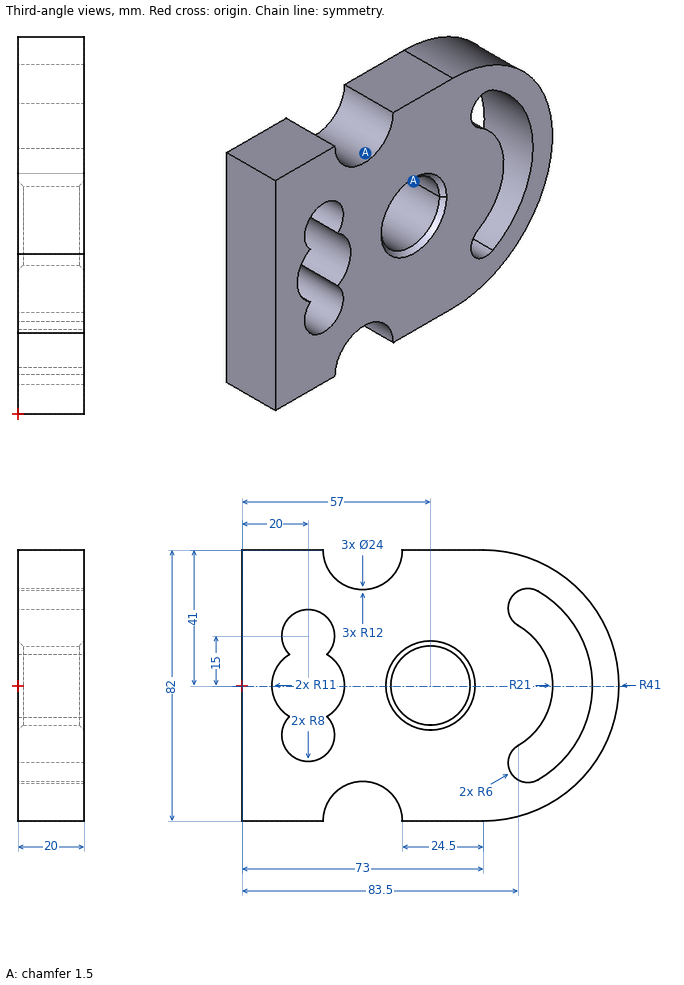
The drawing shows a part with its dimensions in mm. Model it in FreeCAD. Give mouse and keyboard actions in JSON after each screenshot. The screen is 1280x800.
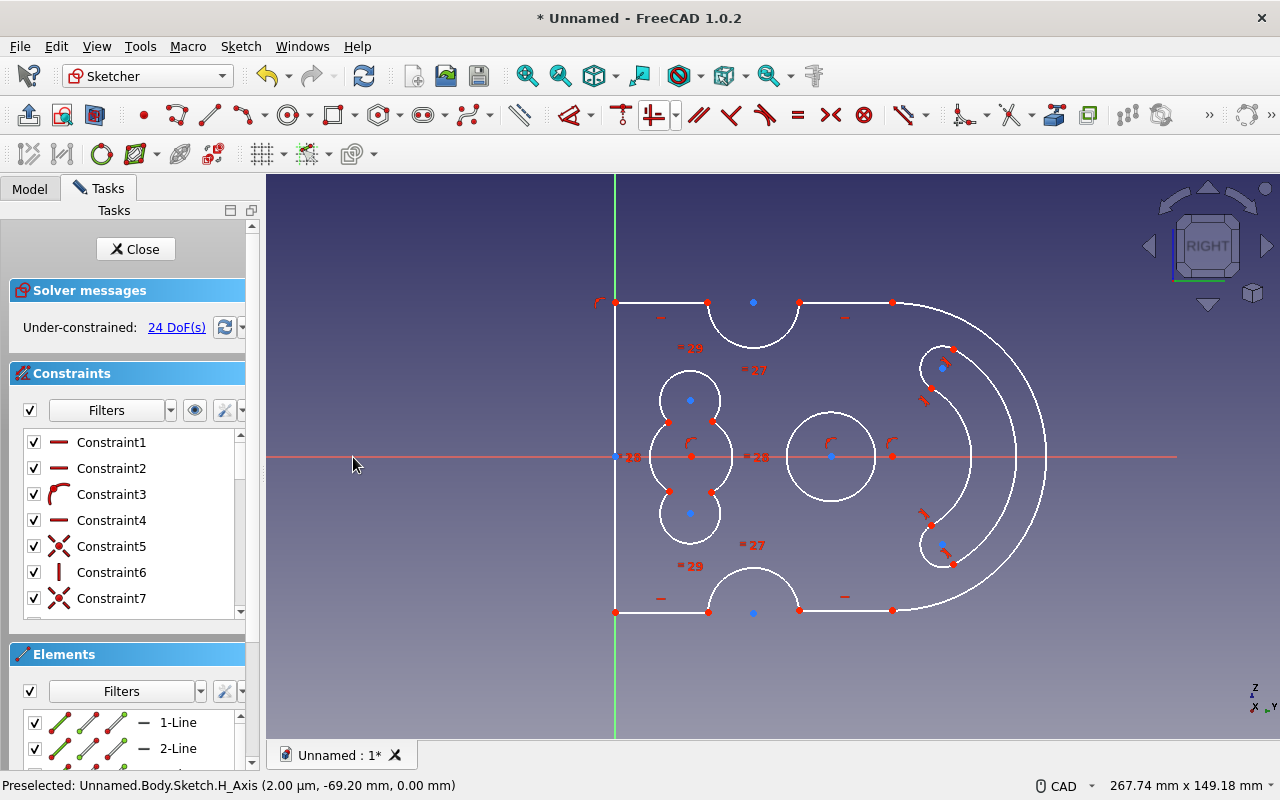
{"action": "left_click", "coordinate": [754, 303]}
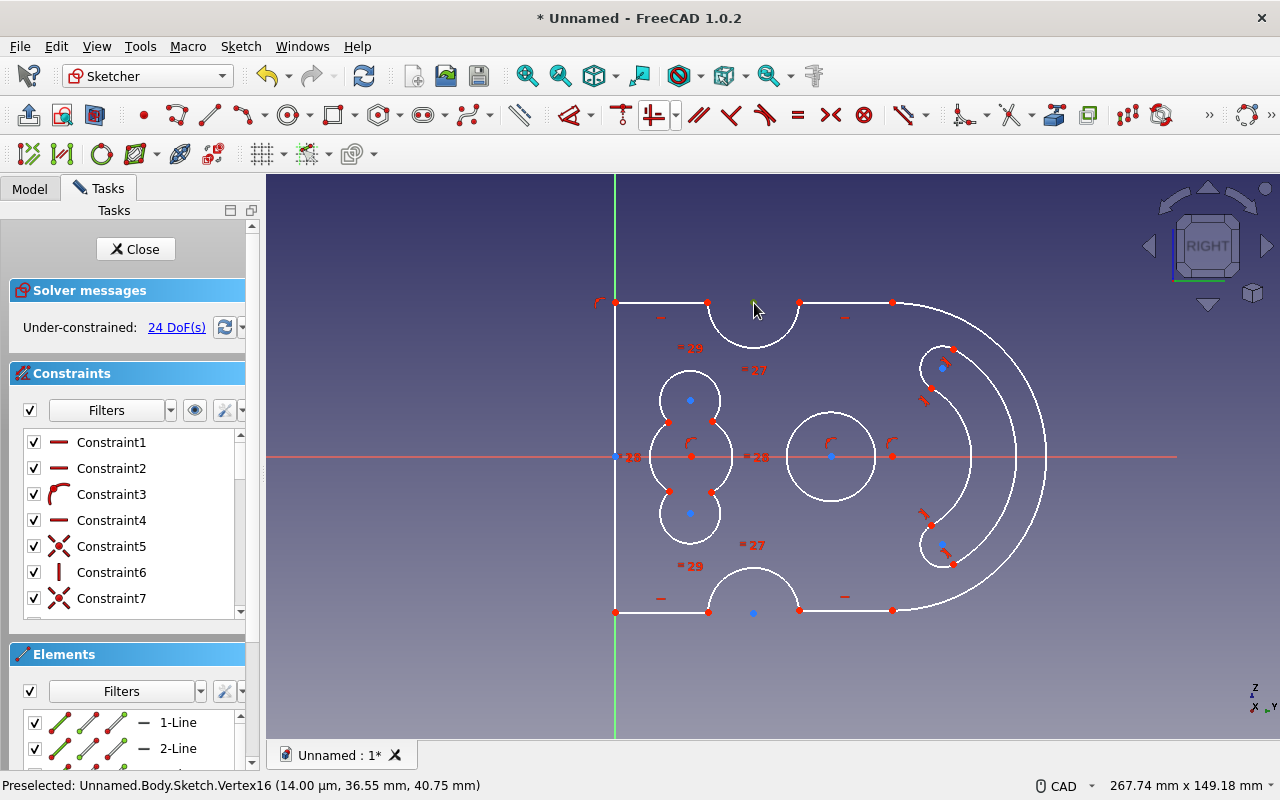
{"action": "left_click", "coordinate": [754, 614]}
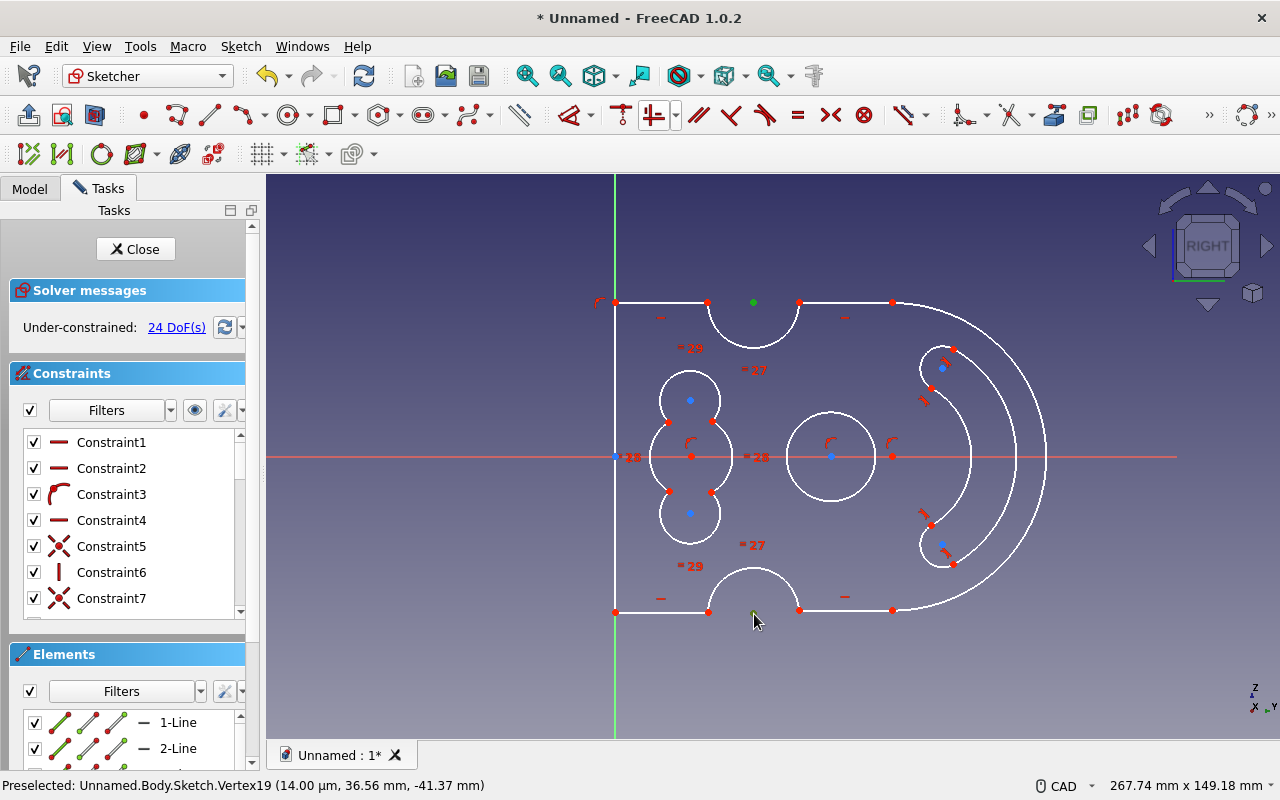
{"action": "left_click", "coordinate": [353, 457]}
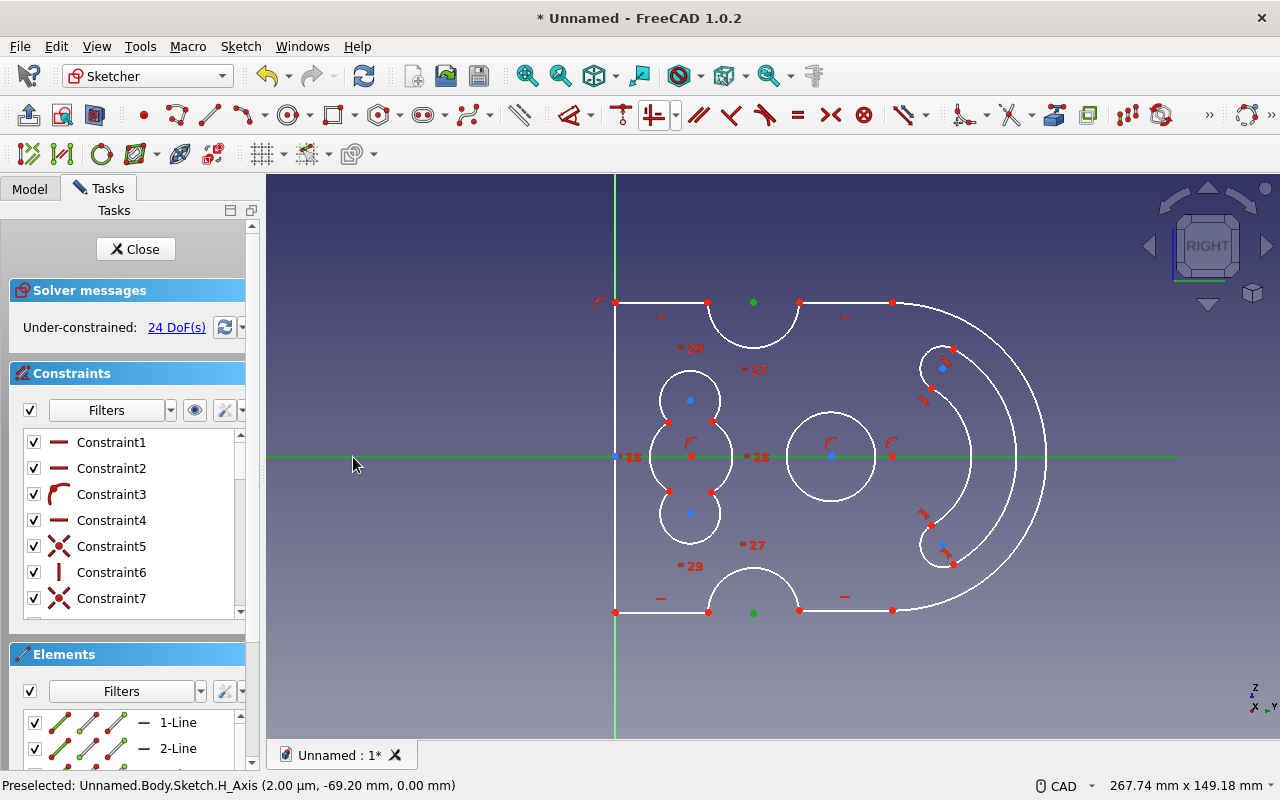
{"action": "left_click", "coordinate": [831, 116]}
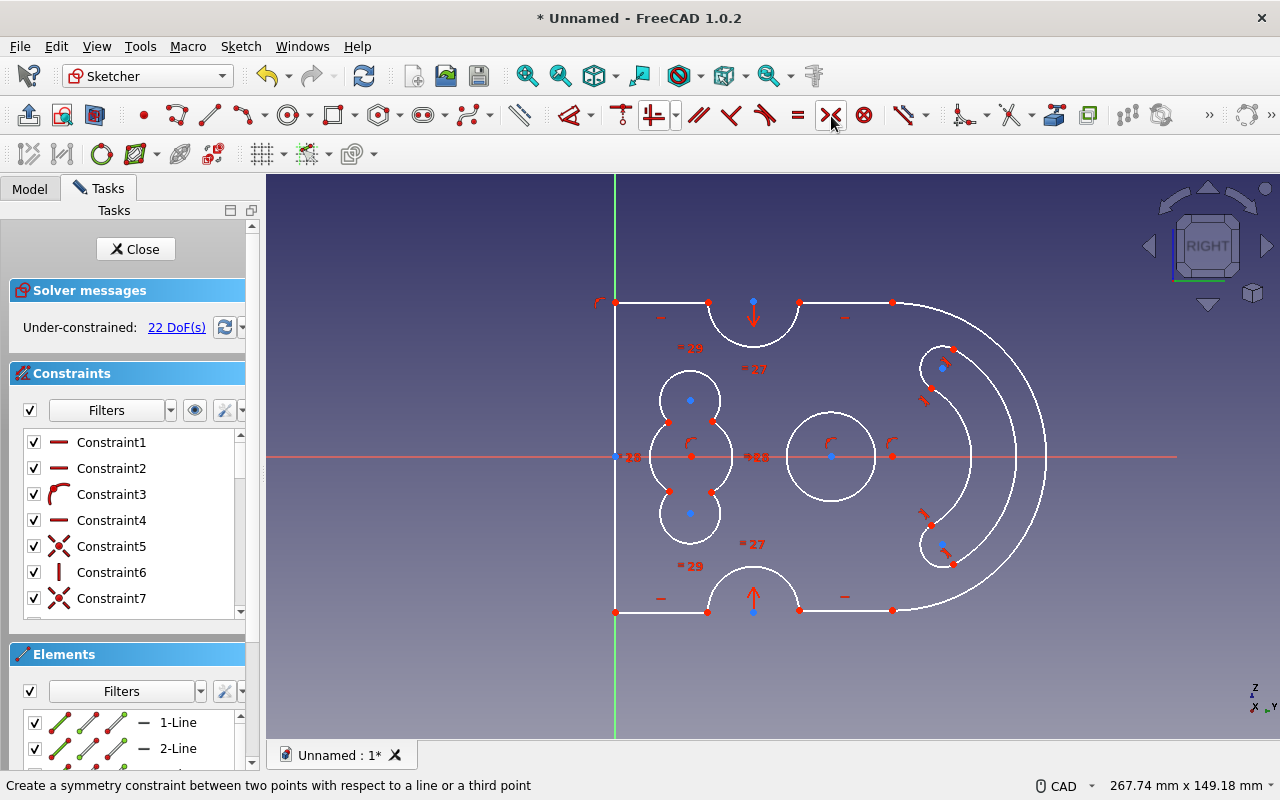
{"action": "left_click", "coordinate": [690, 401]}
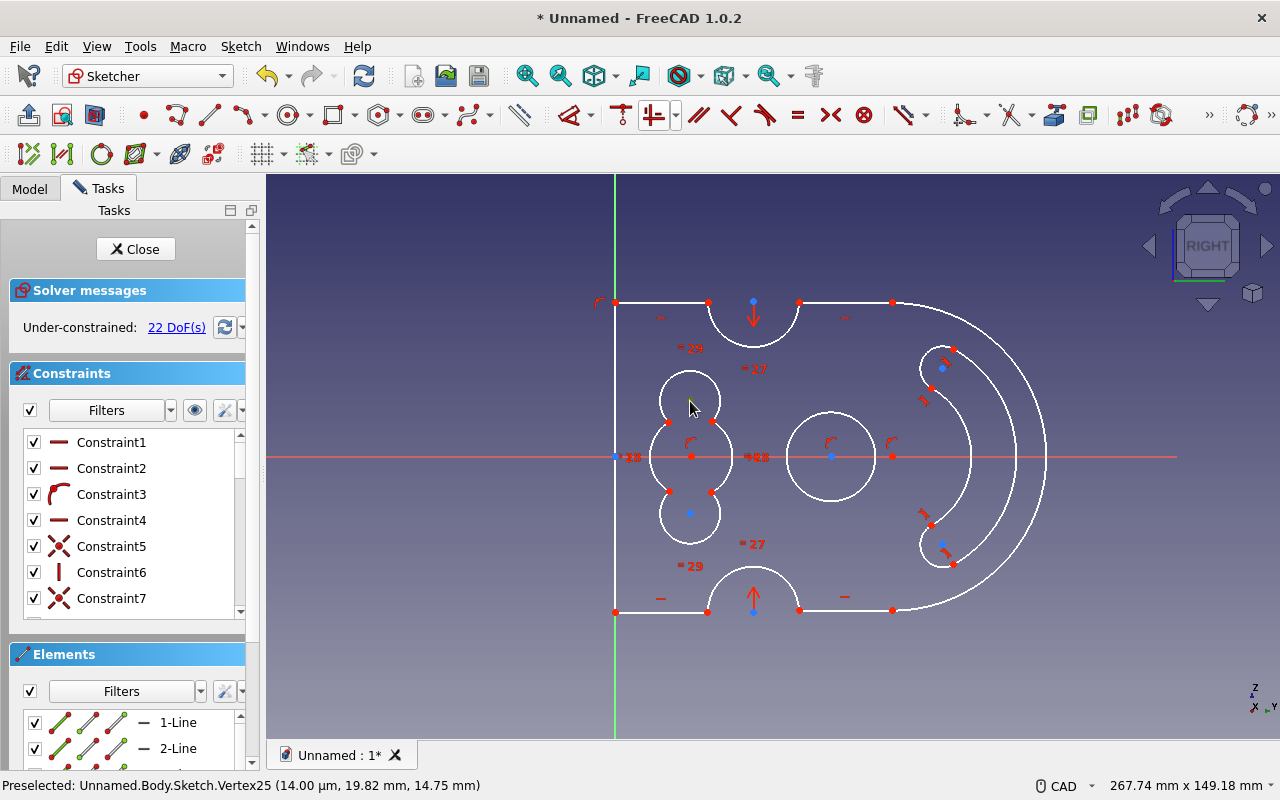
{"action": "left_click", "coordinate": [690, 514]}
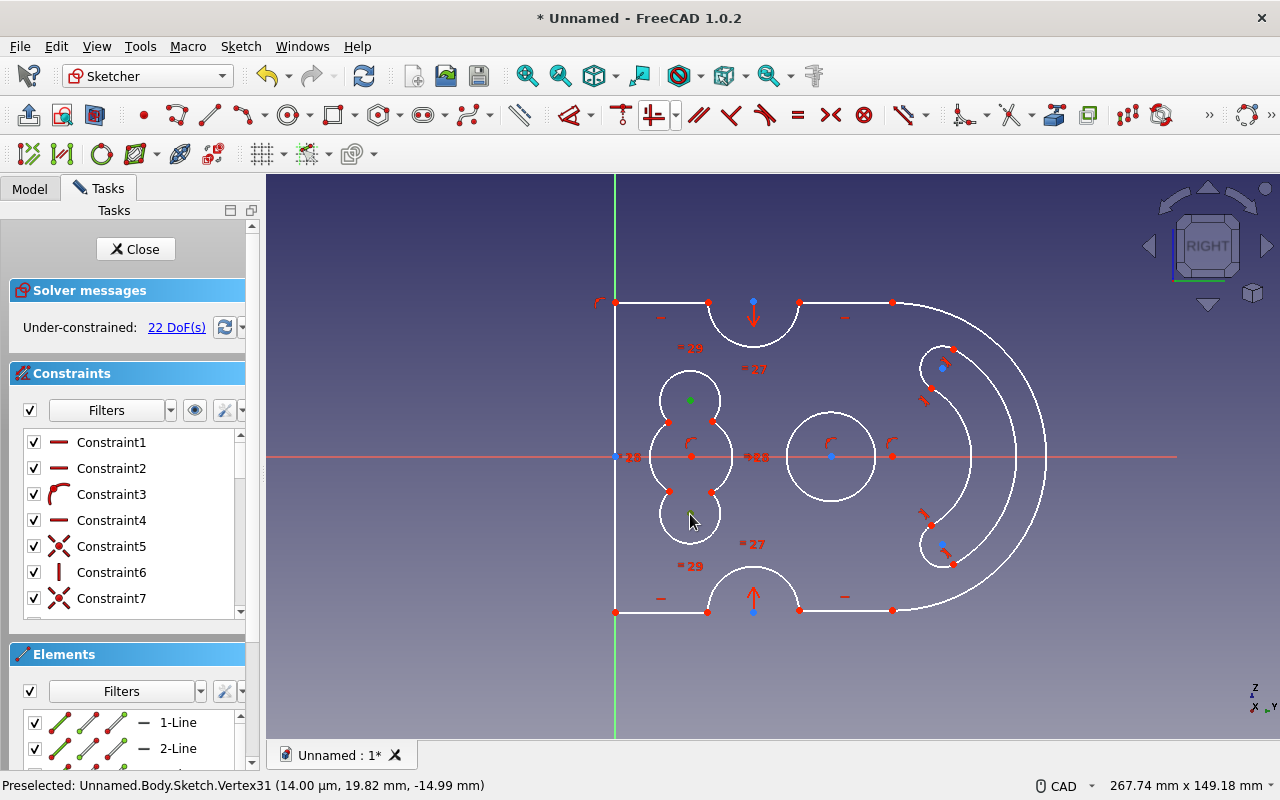
{"action": "left_click", "coordinate": [353, 457]}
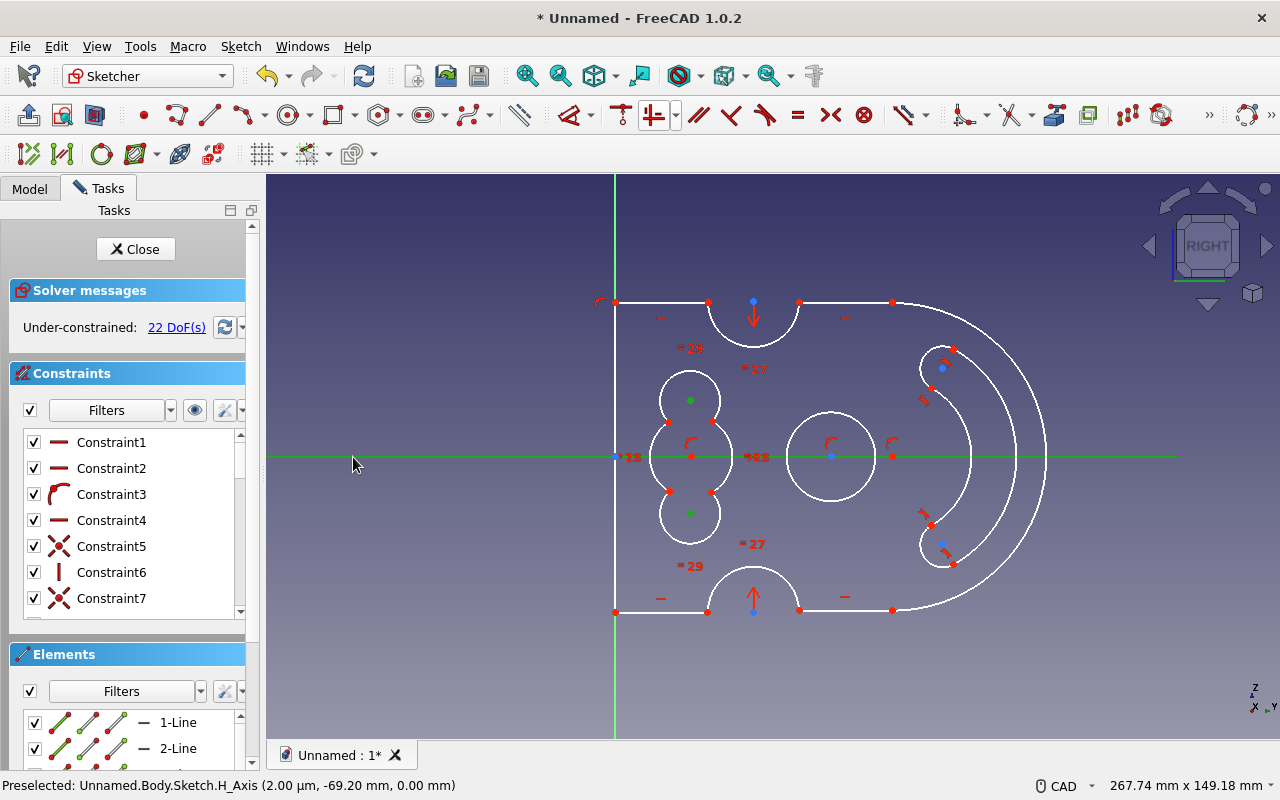
{"action": "key", "text": "s"}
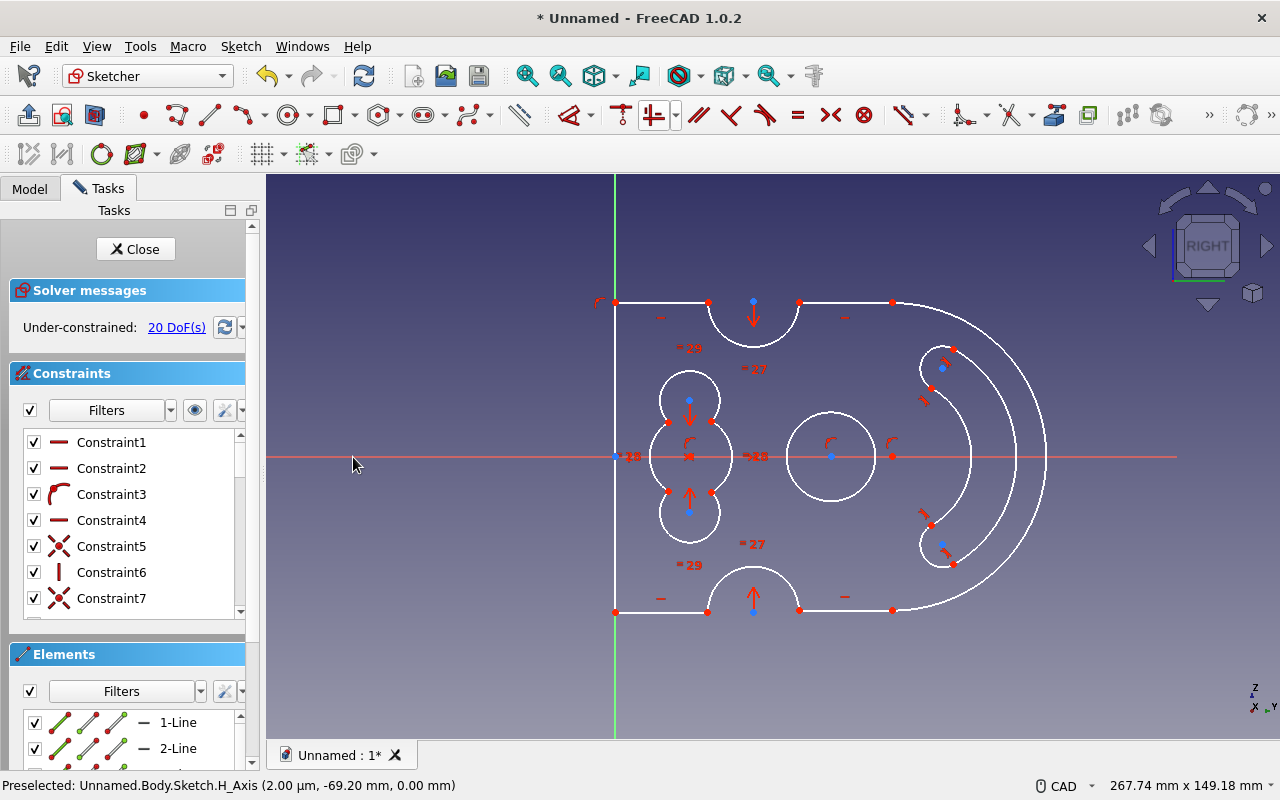
{"action": "left_click", "coordinate": [1017, 547]}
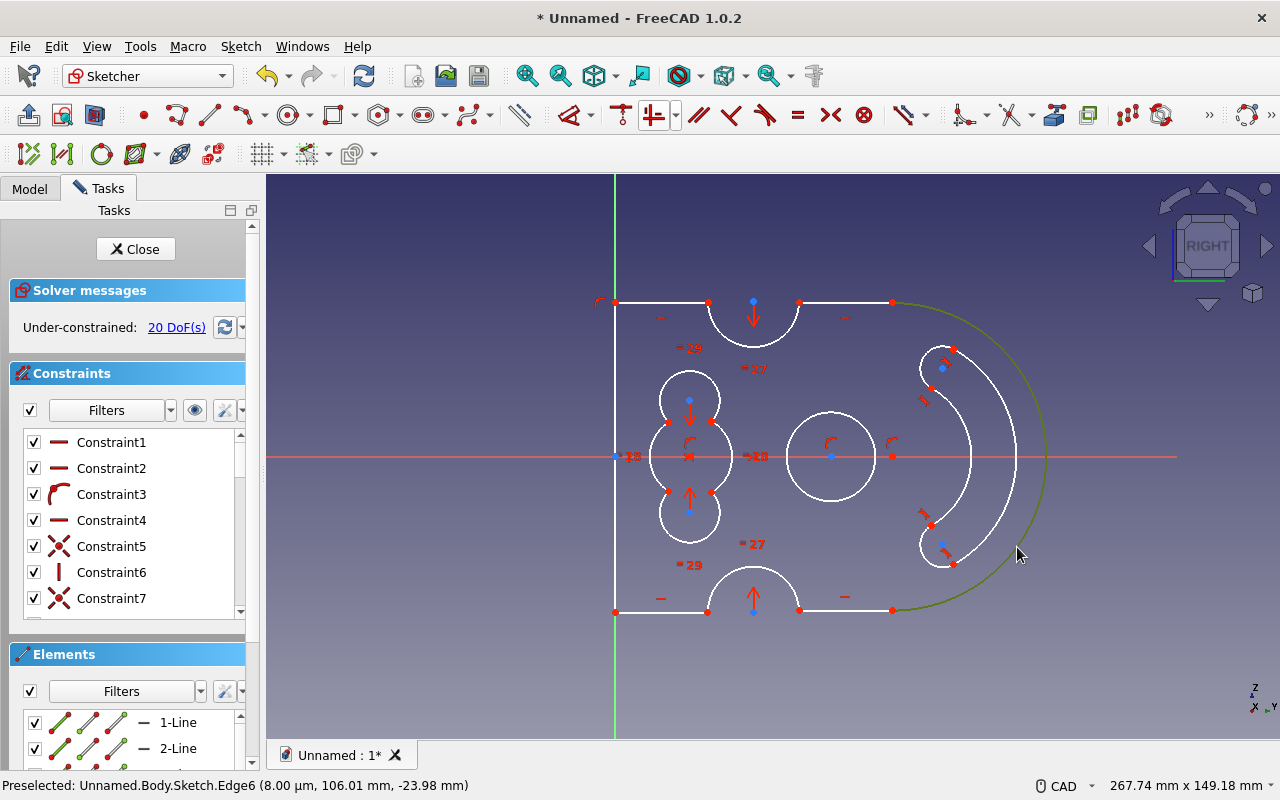
{"action": "key", "text": "k r"}